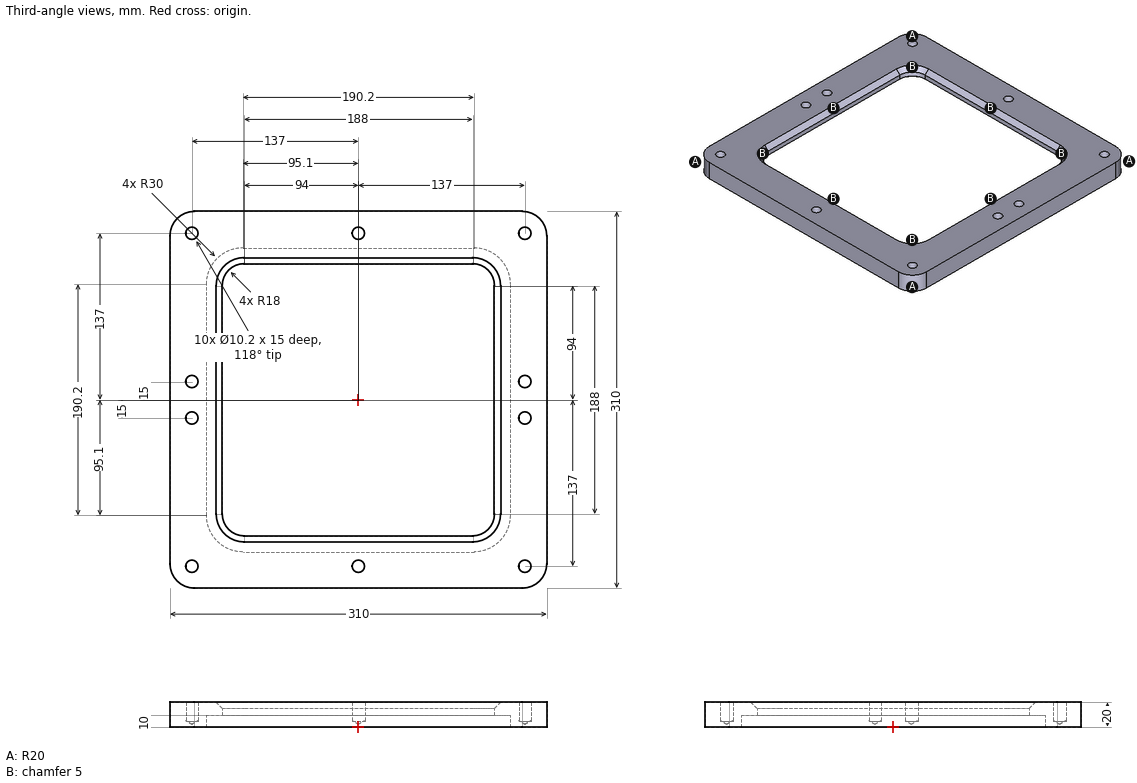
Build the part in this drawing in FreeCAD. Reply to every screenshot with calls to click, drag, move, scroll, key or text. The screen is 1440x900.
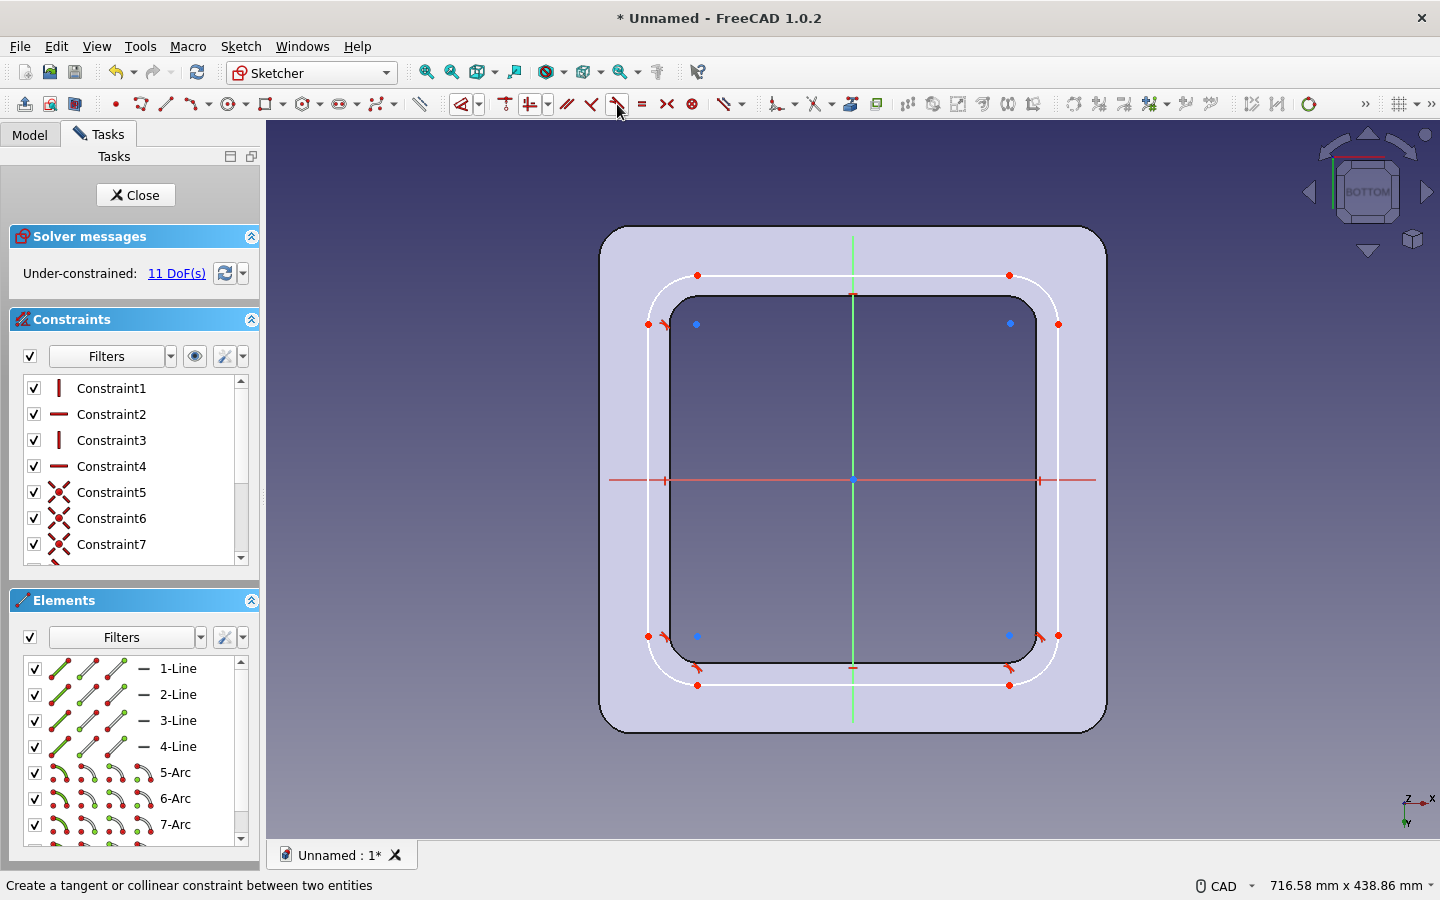
click(1058, 543)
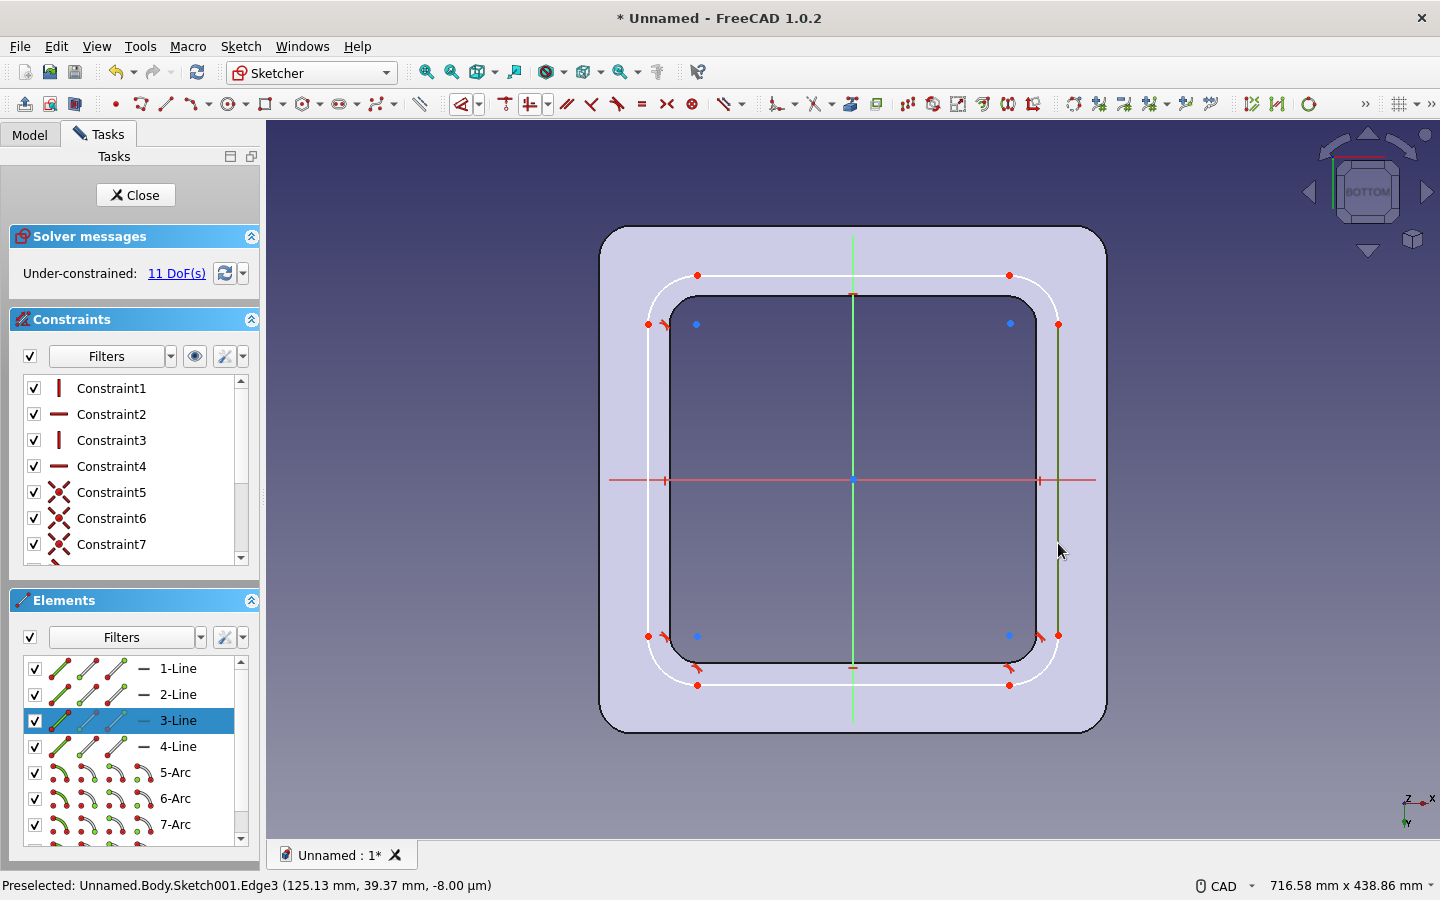
click(1053, 303)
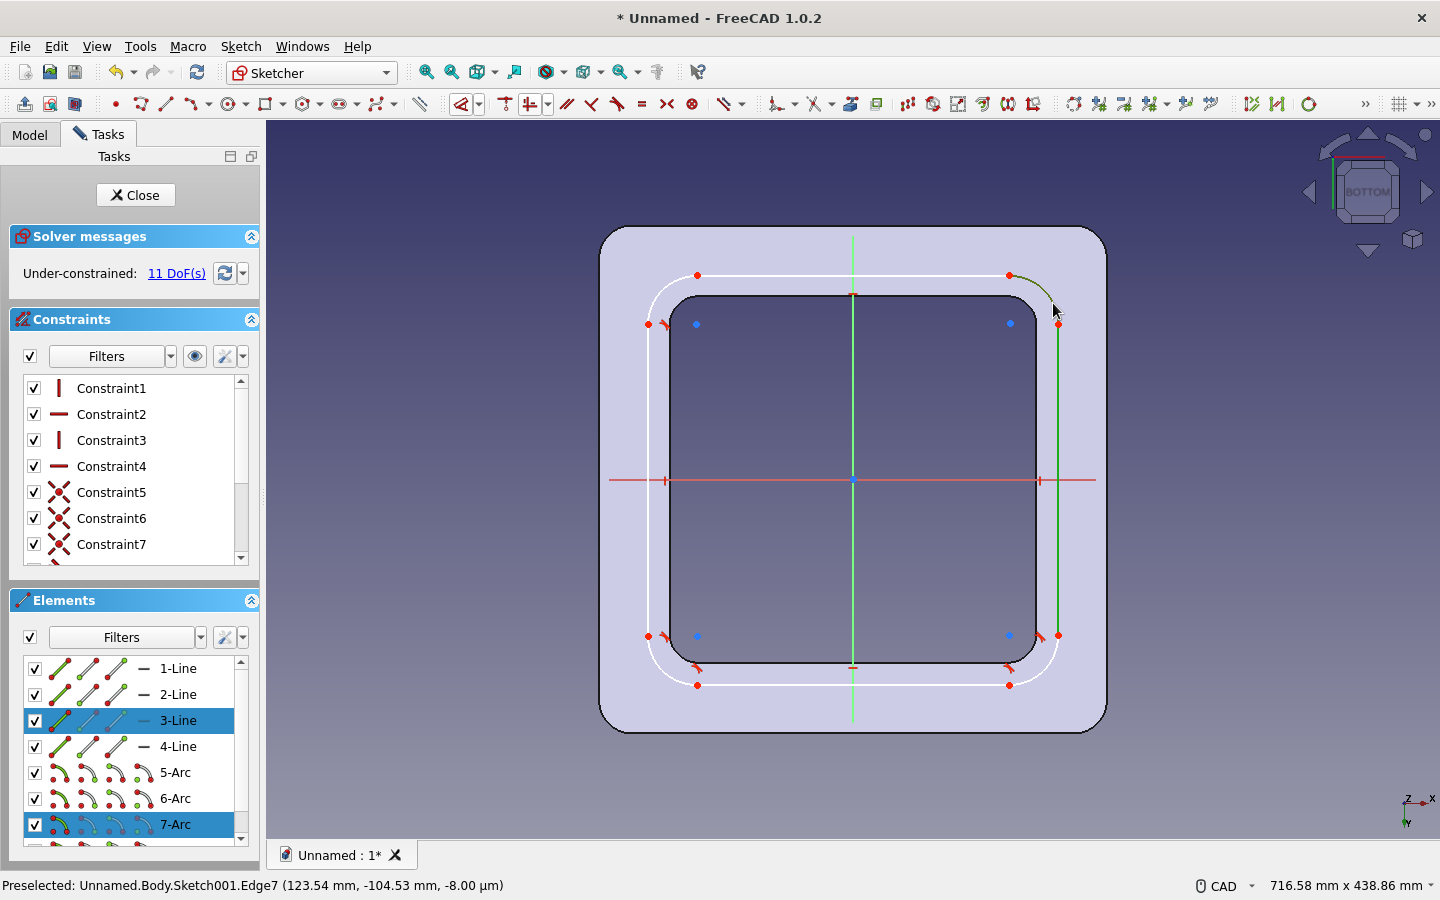
click(617, 104)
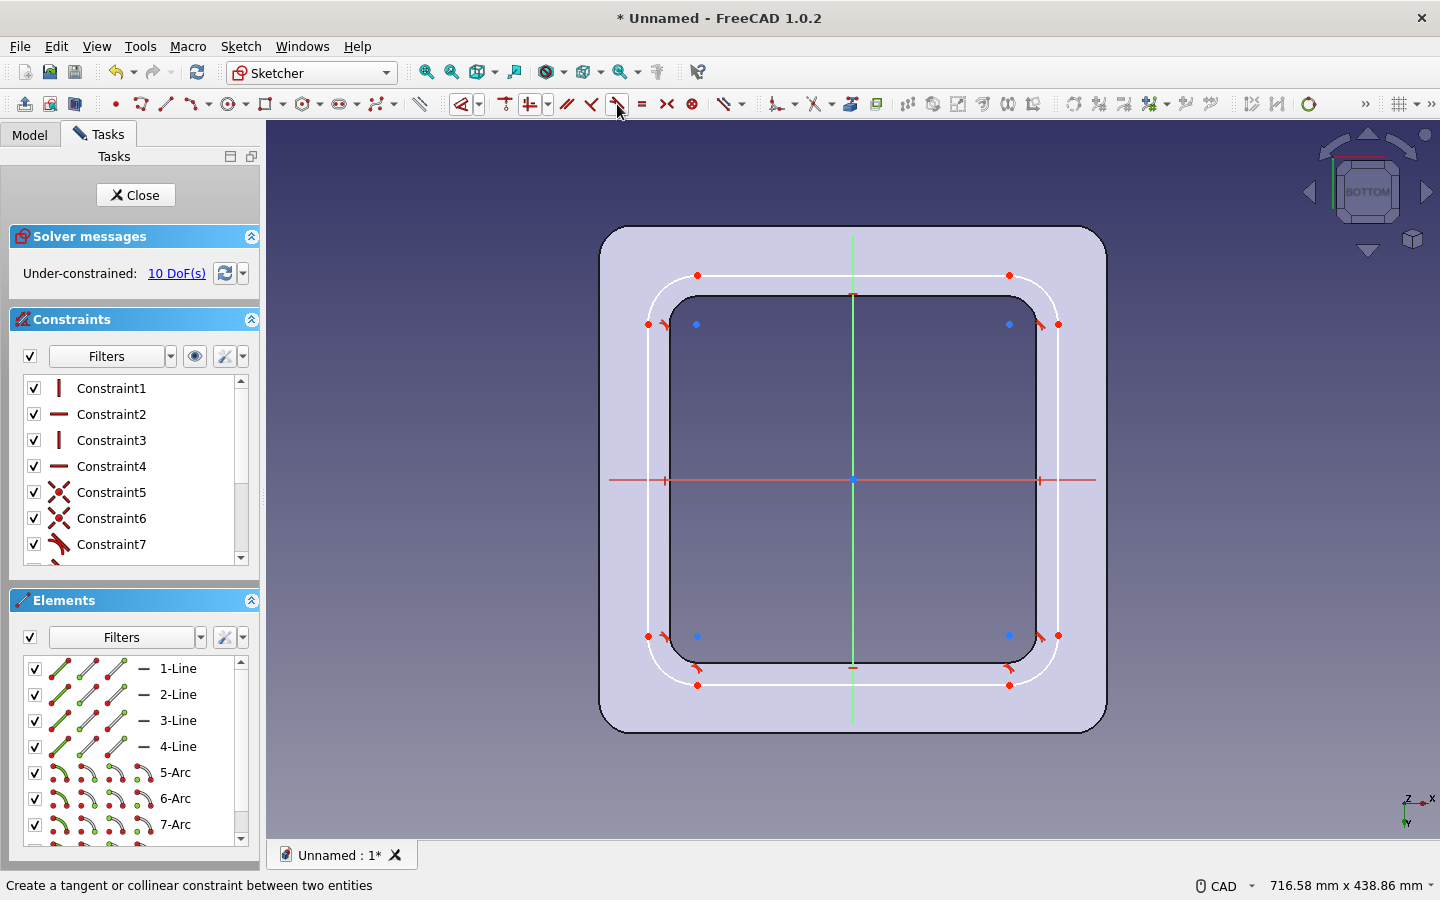
click(915, 276)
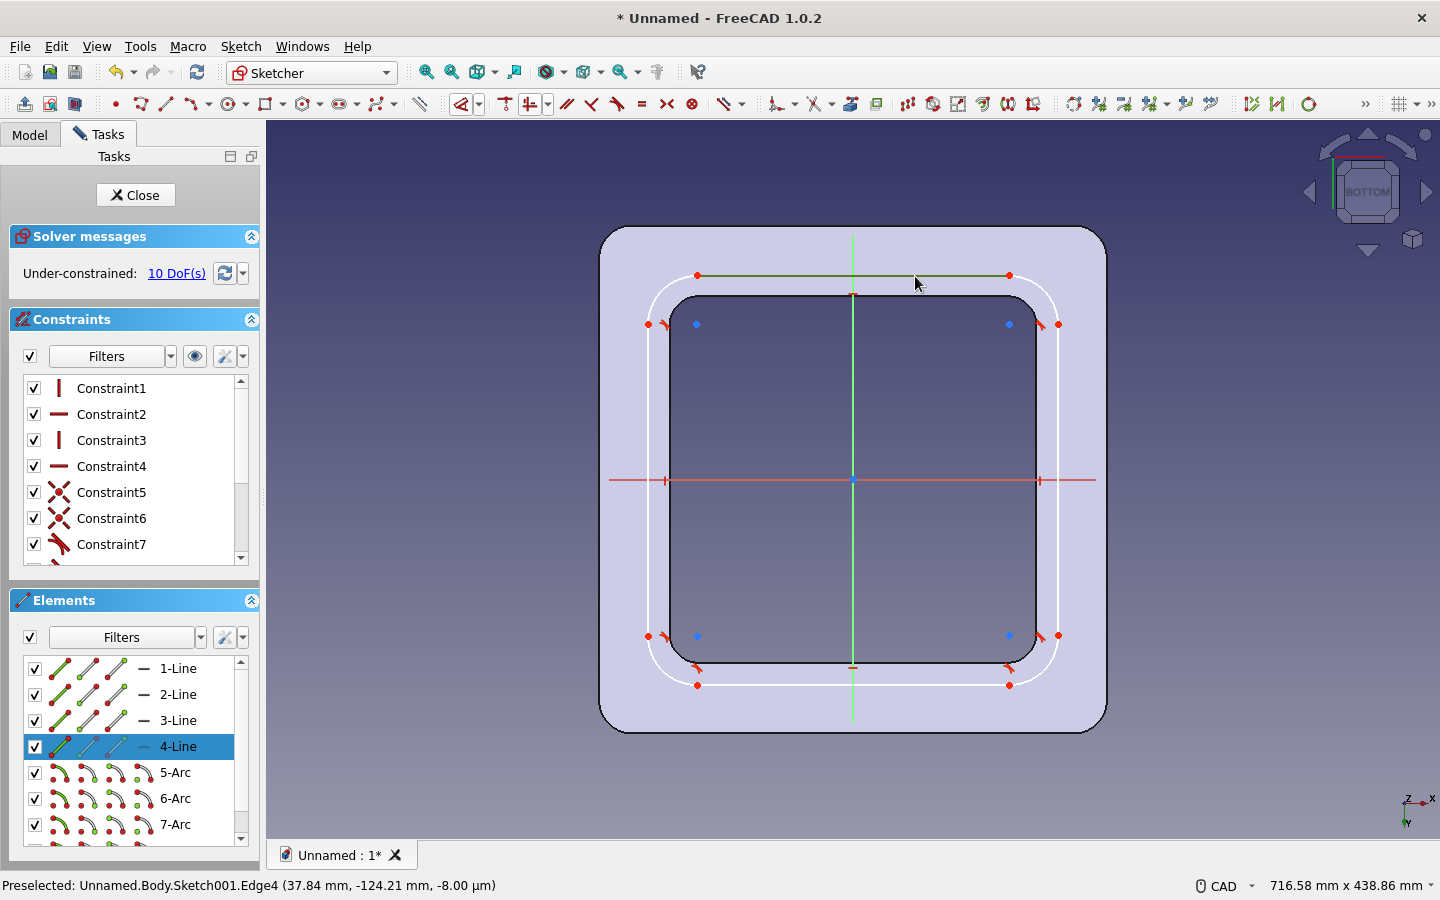
click(1053, 303)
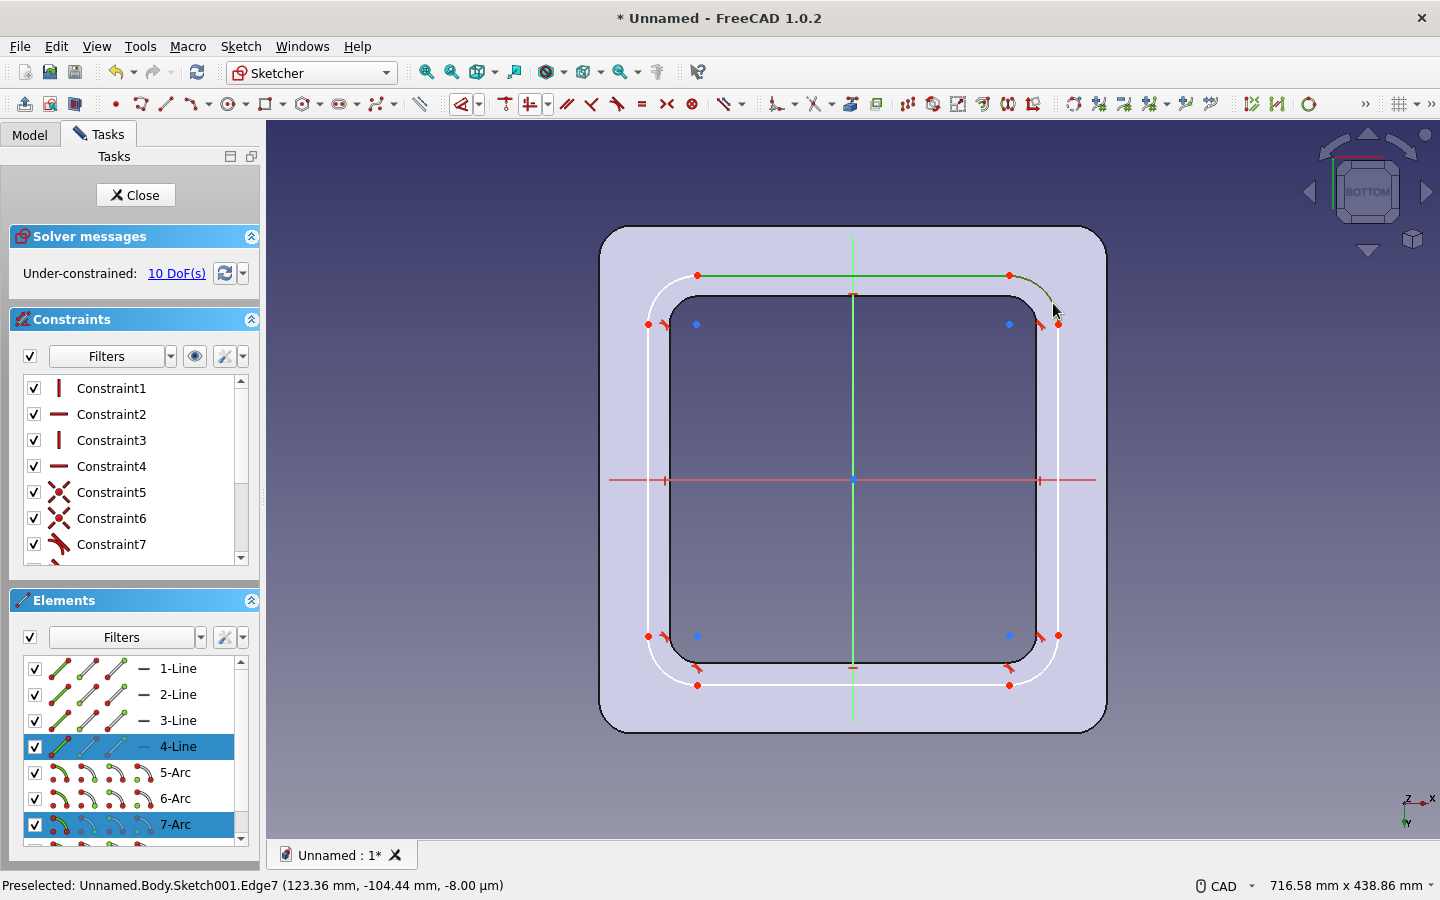
click(617, 104)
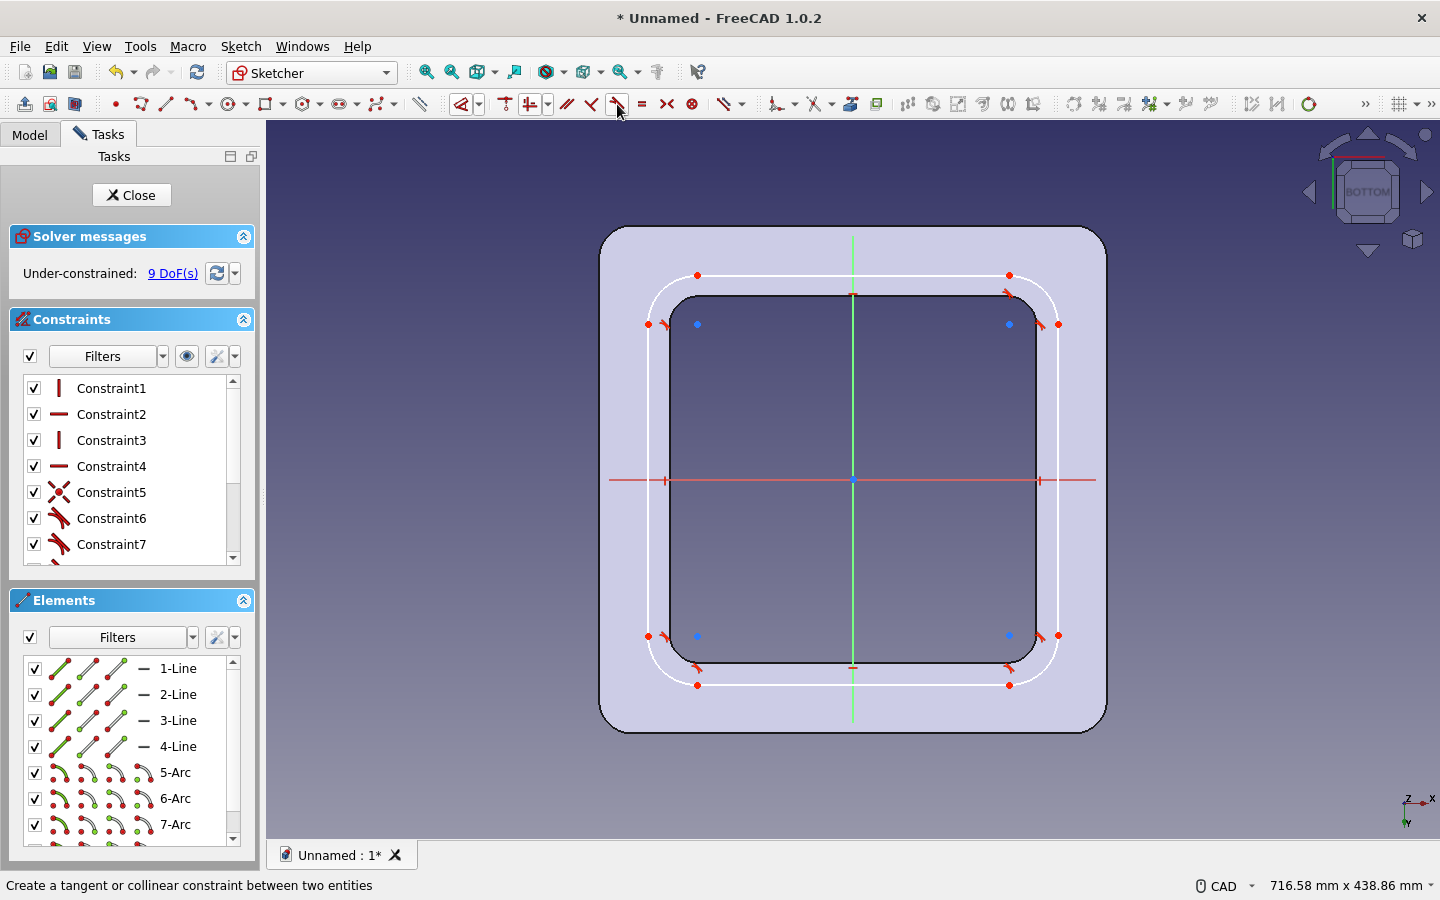
click(915, 276)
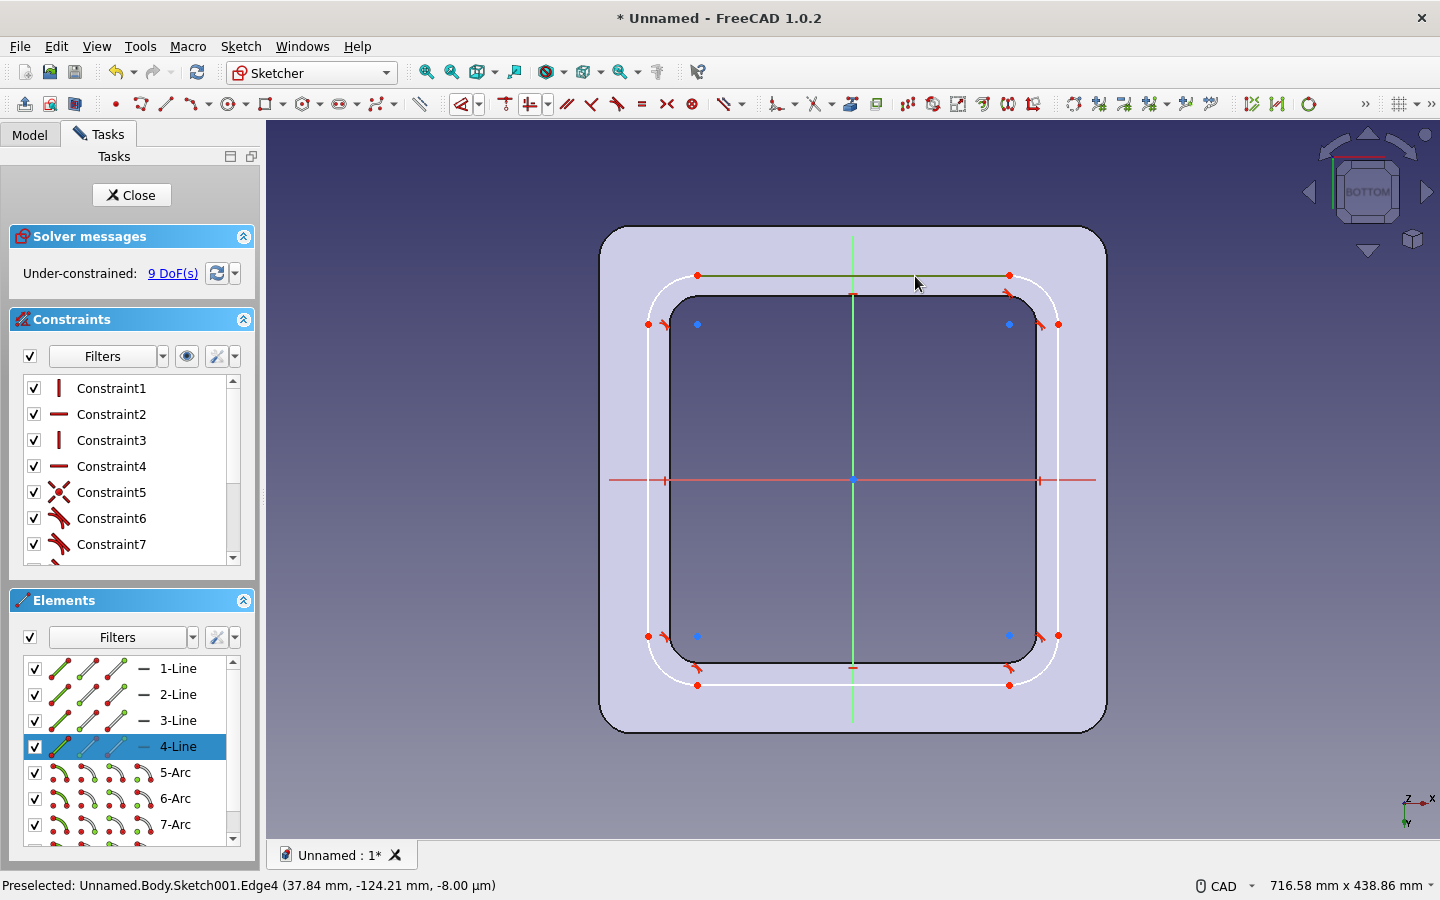
click(675, 281)